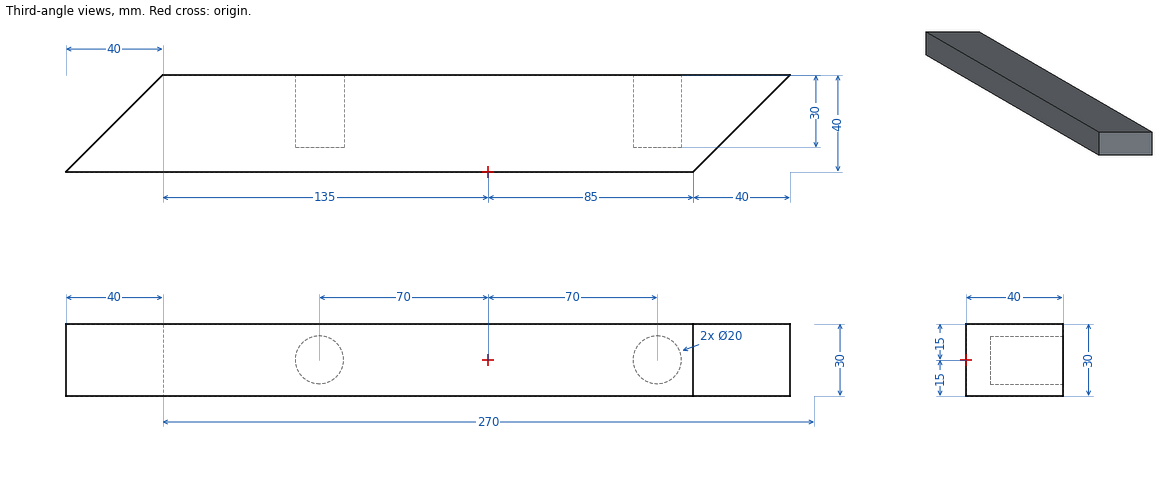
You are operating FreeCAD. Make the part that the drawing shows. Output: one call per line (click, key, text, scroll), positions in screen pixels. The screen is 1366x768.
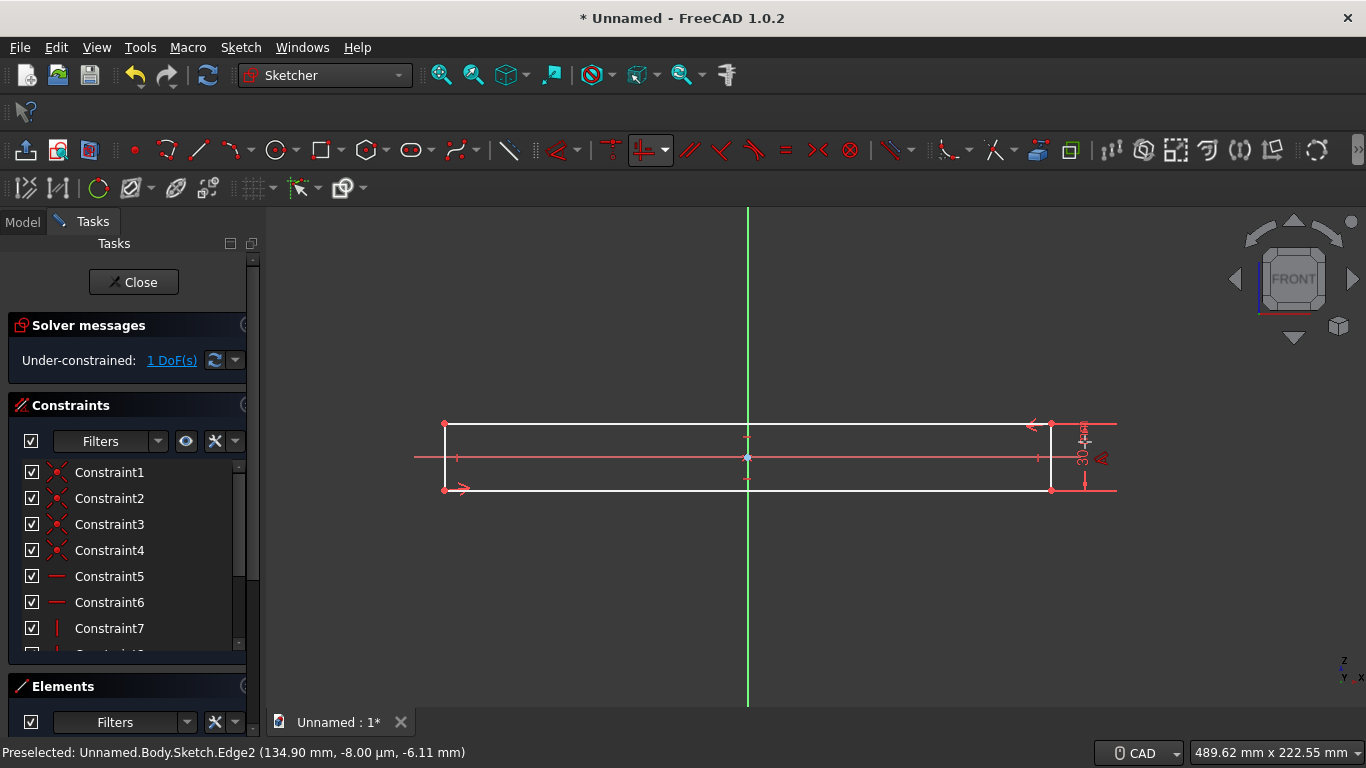
click(627, 491)
click(609, 525)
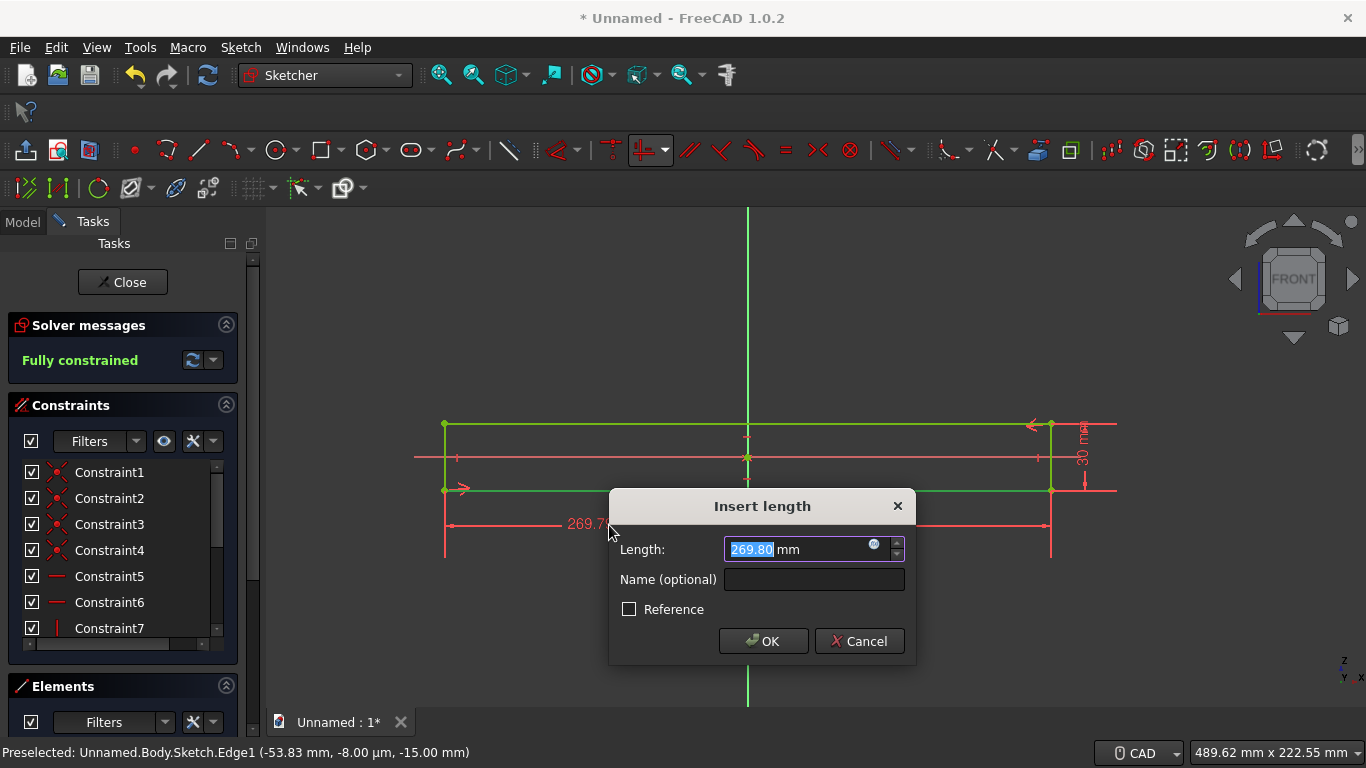
text(270)
key(Return)
key(Escape)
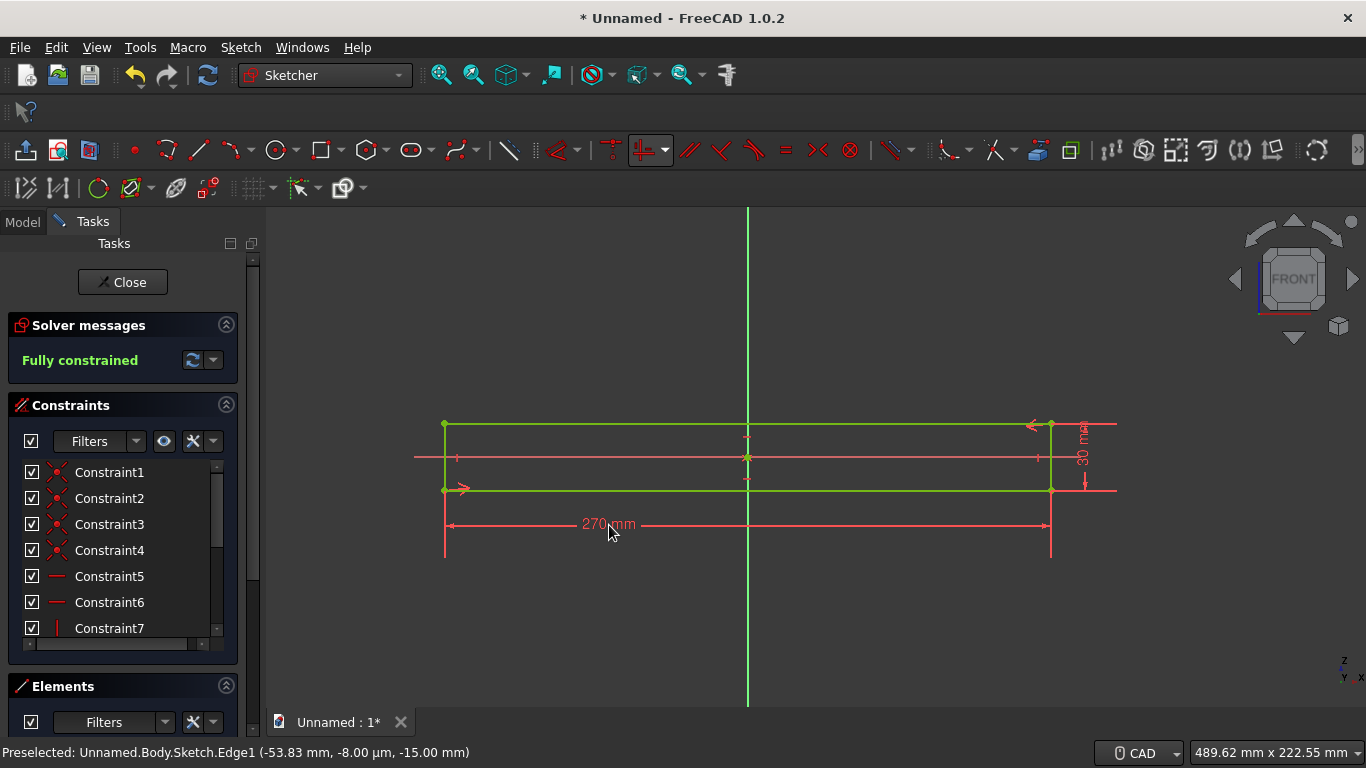
click(123, 282)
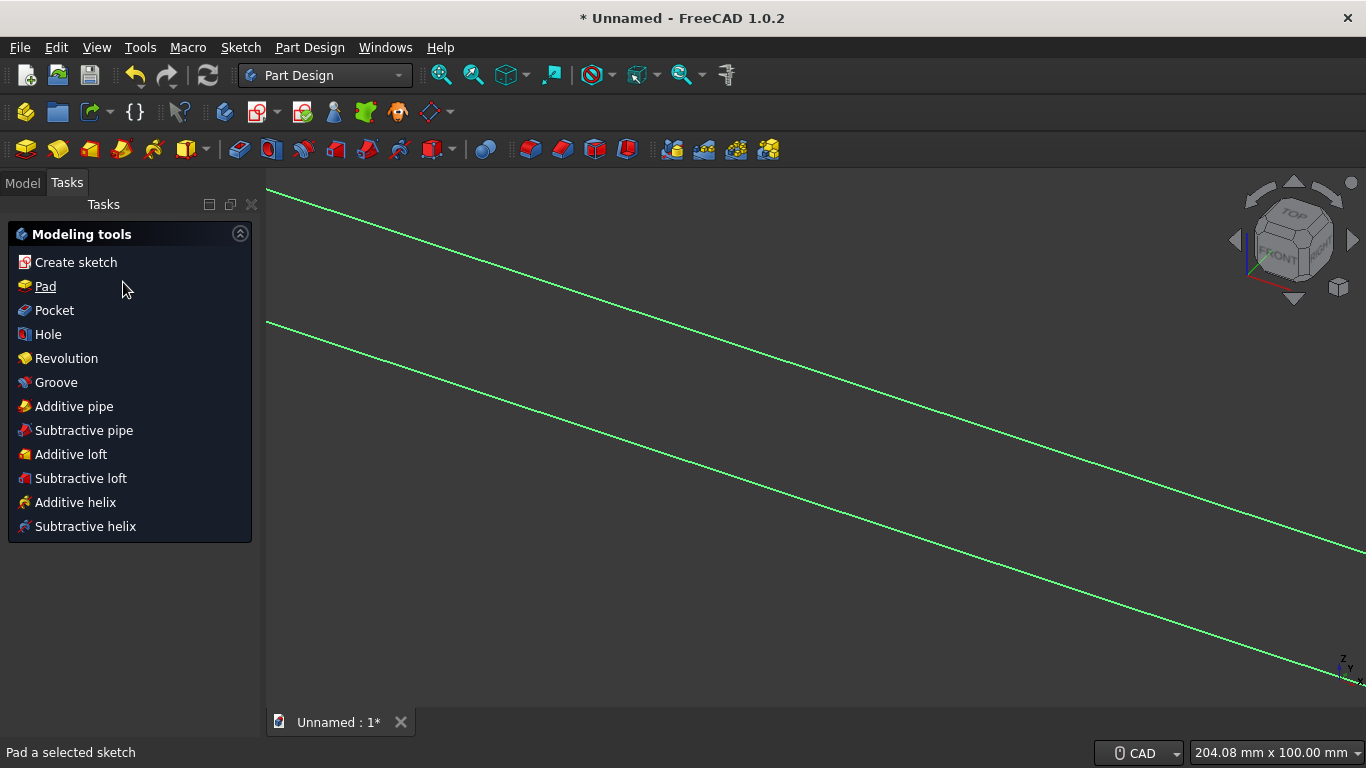
click(26, 150)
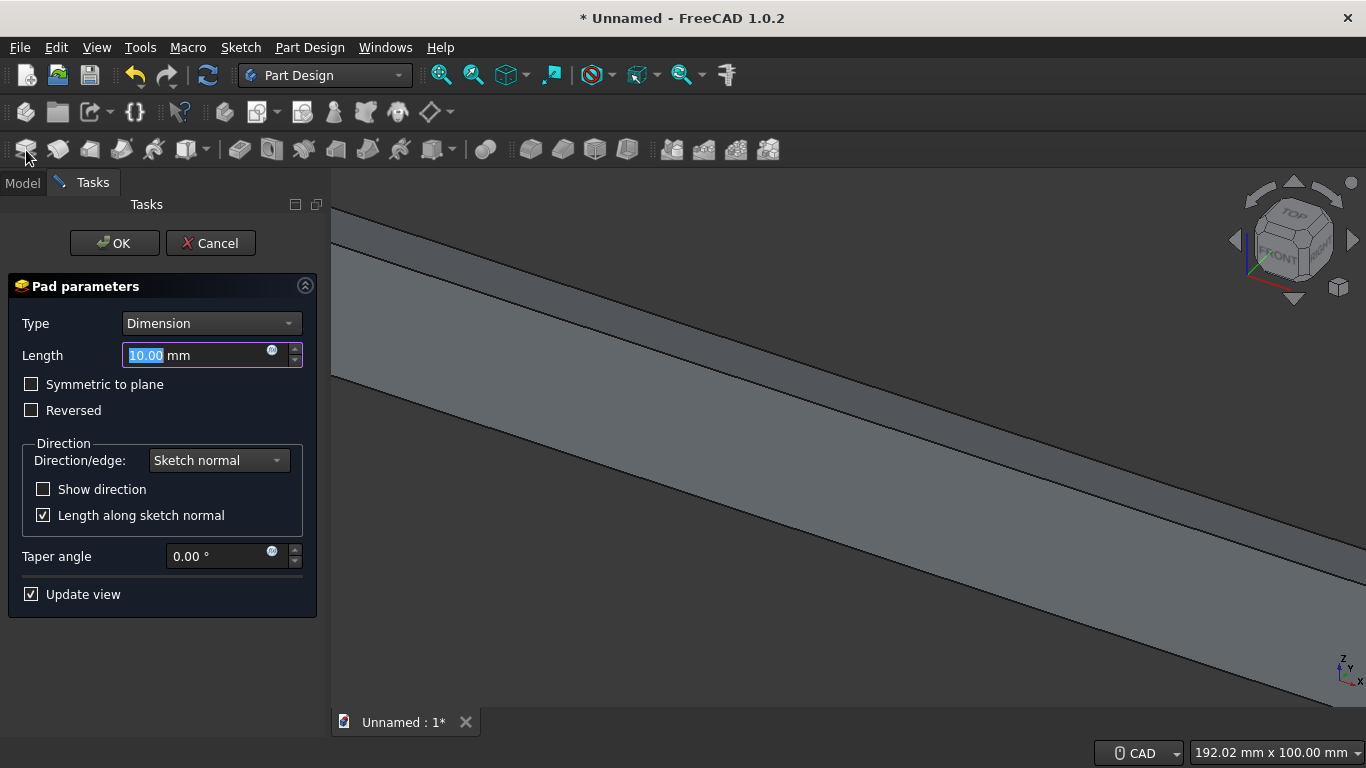
text(40)
key(Tab)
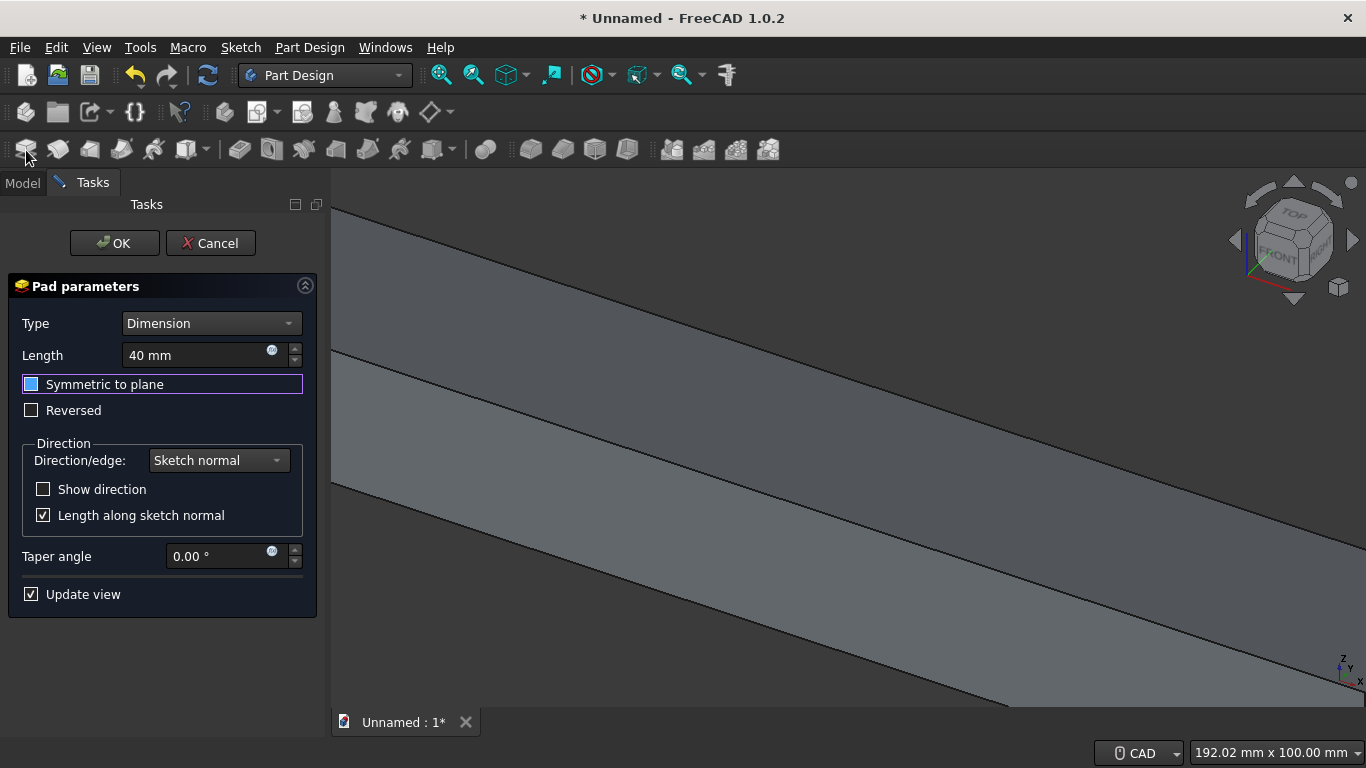
click(30, 410)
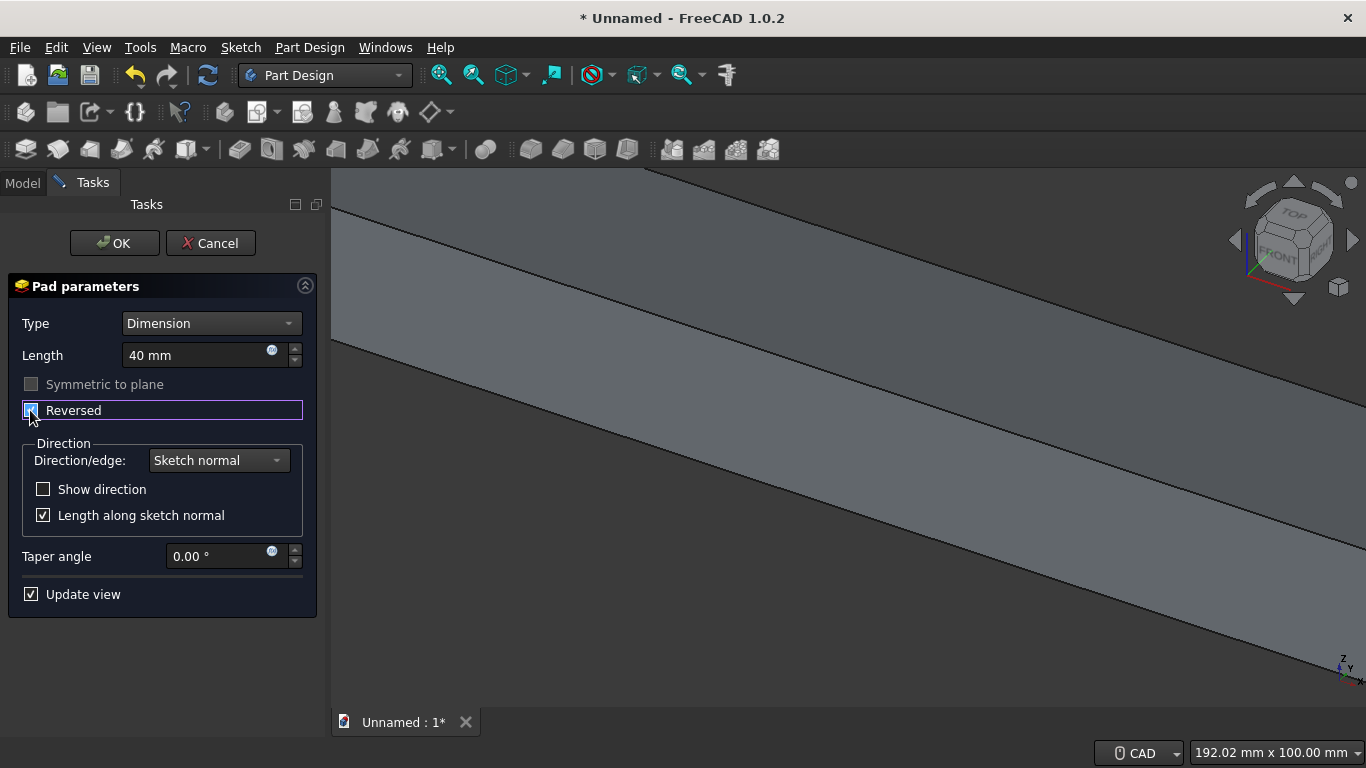
click(115, 243)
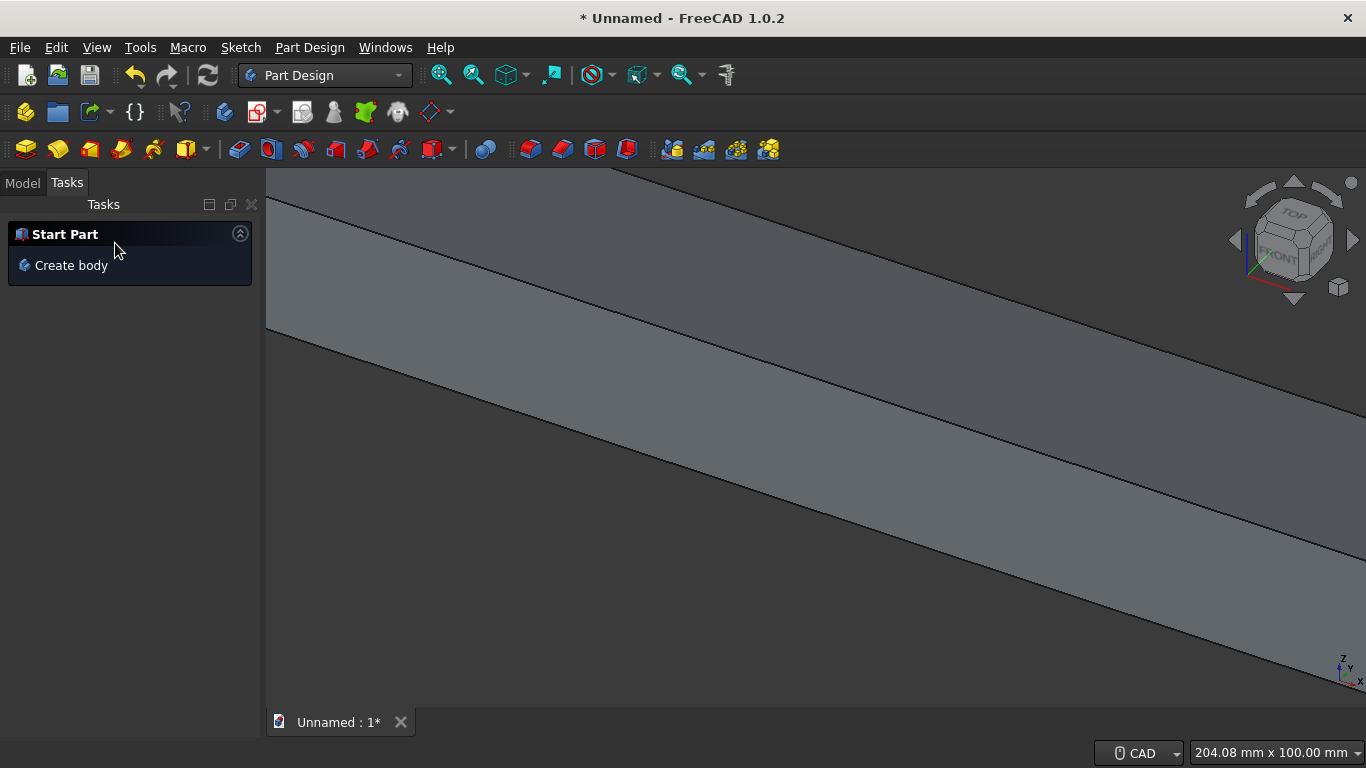
key(v)
key(f)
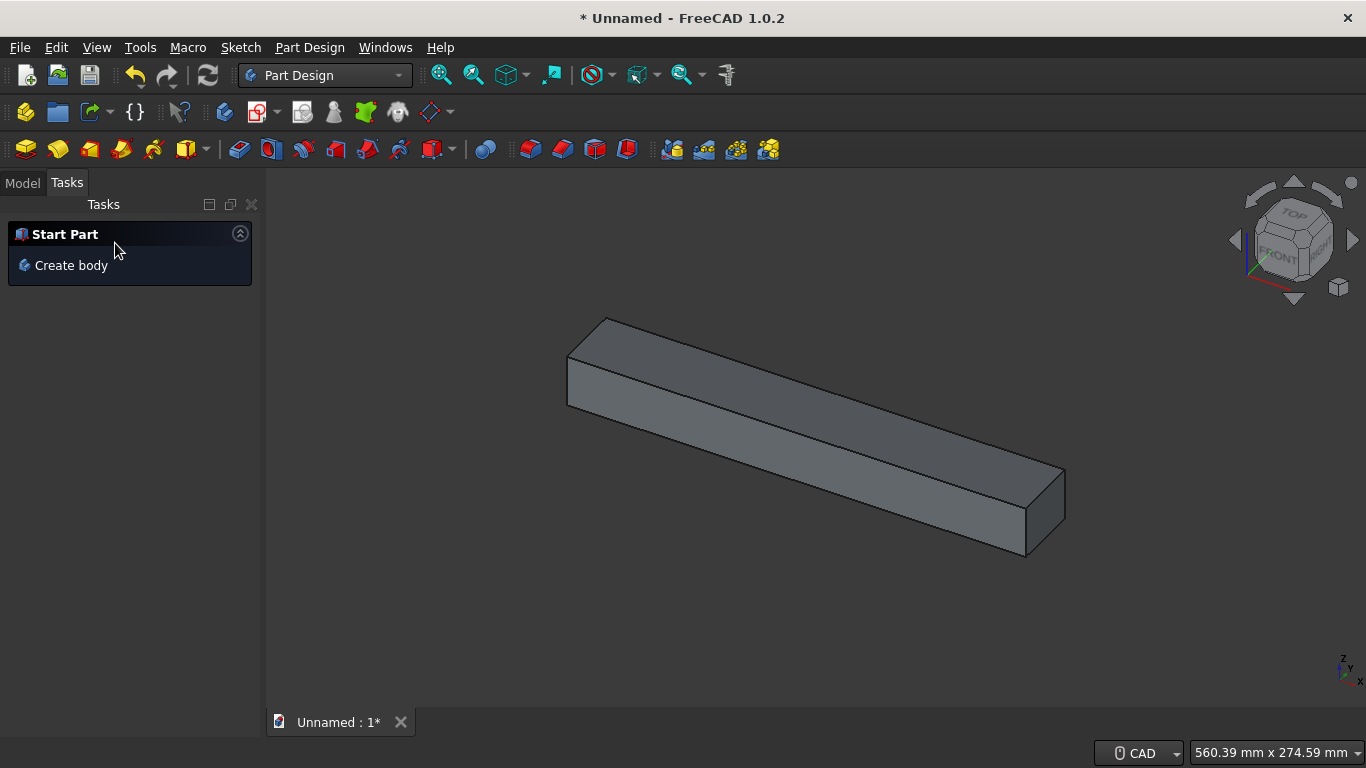
key(4)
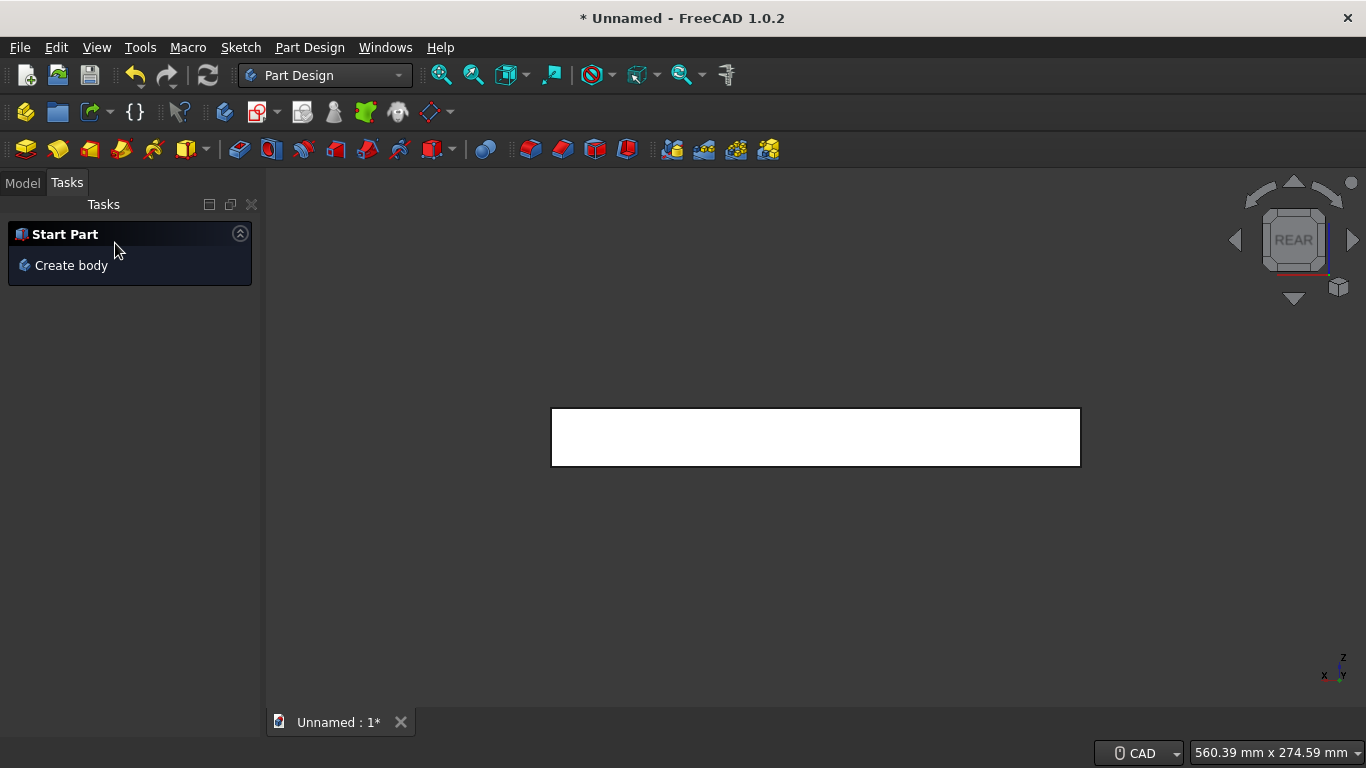
click(589, 437)